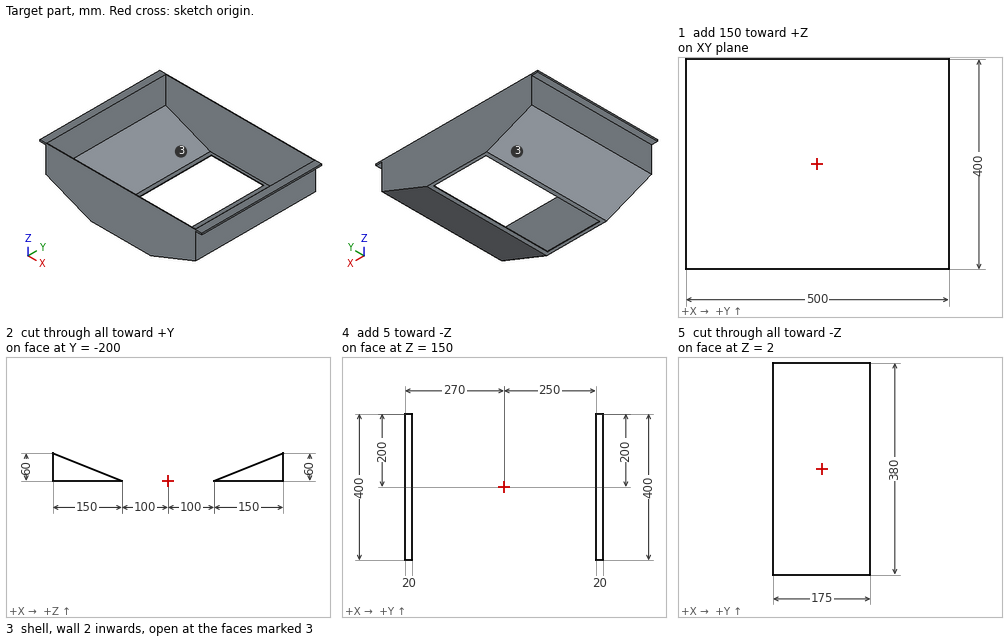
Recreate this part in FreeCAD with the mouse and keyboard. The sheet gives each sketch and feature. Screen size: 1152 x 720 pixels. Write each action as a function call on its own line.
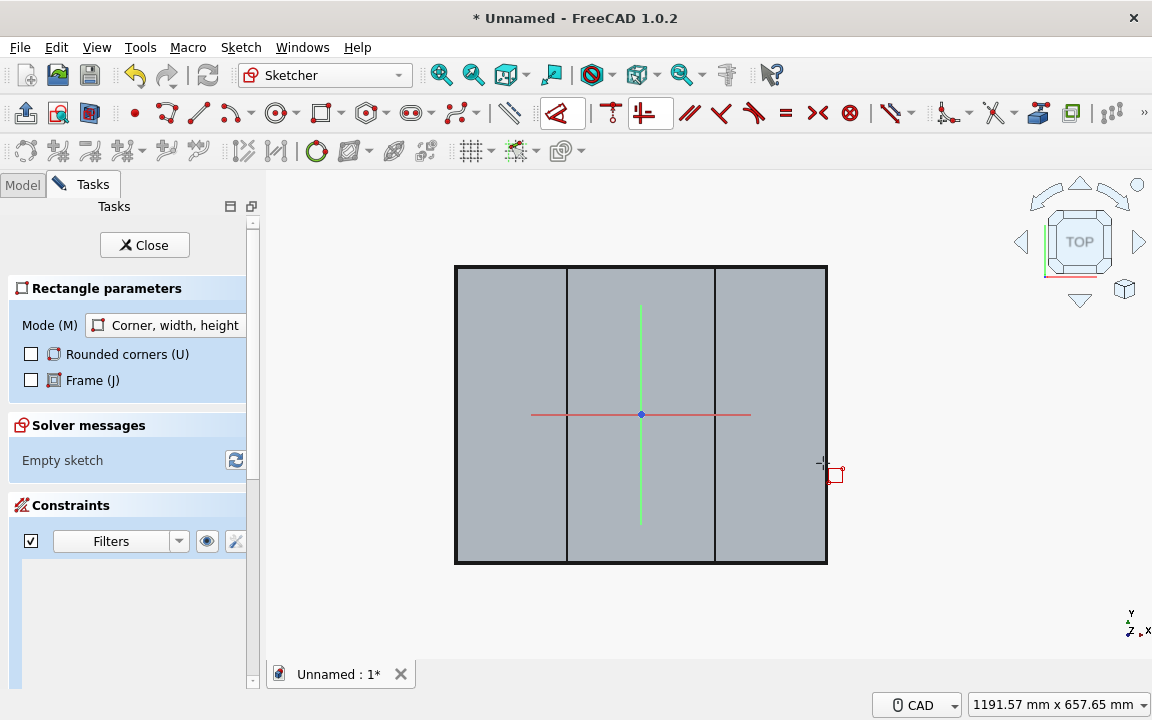
click(441, 266)
click(455, 564)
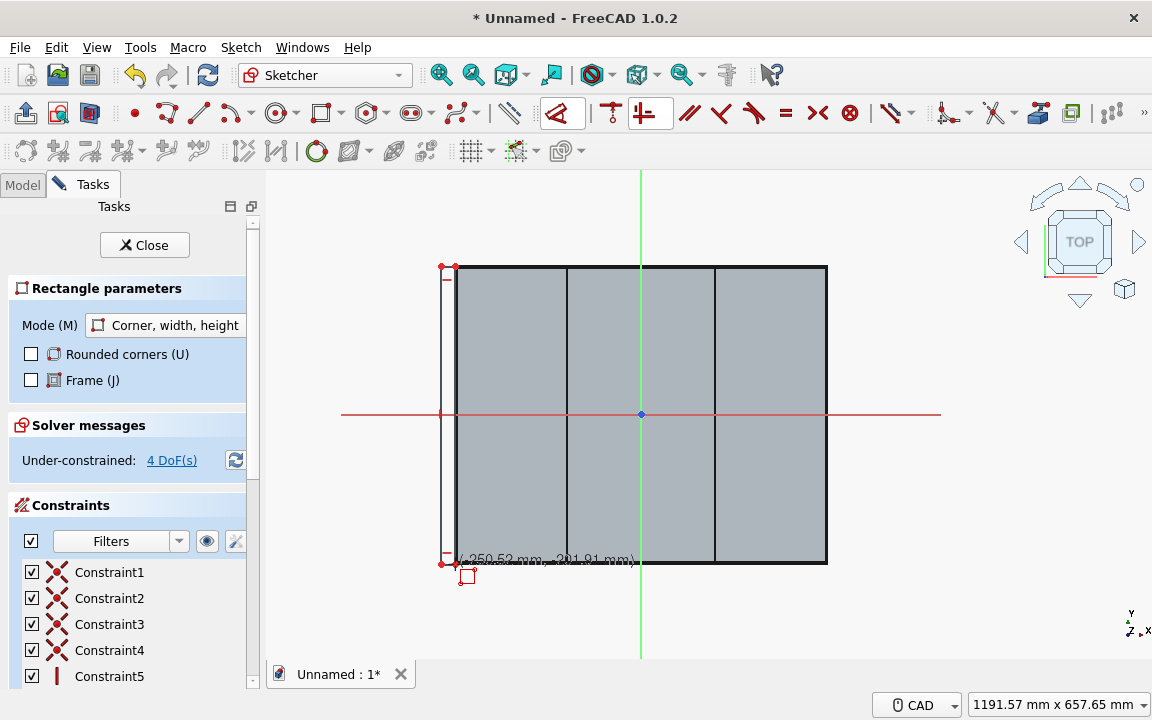
click(827, 266)
click(842, 564)
key(Escape)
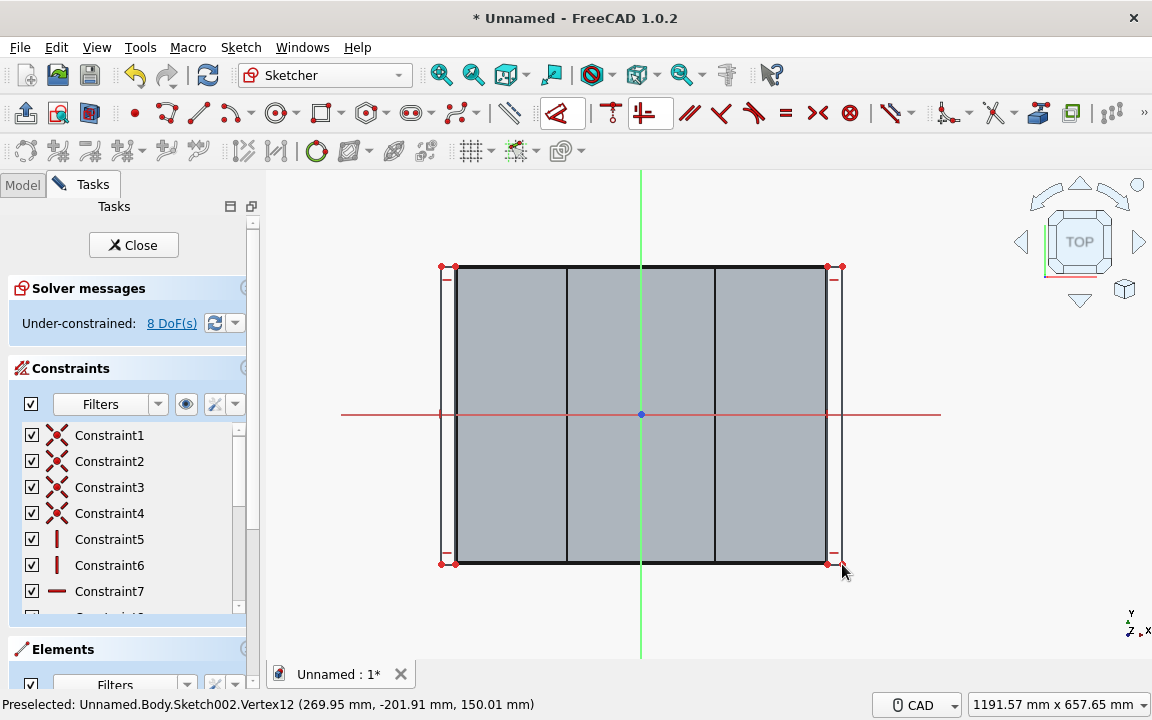
scroll(448, 565, up, 5)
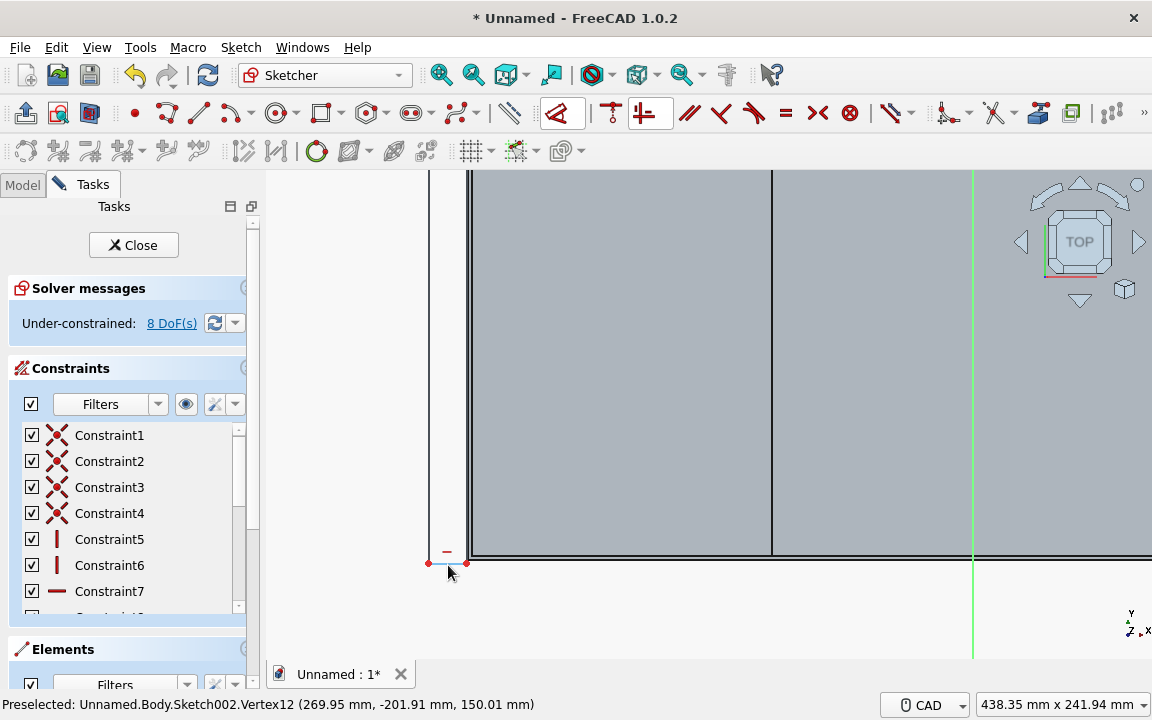
click(448, 564)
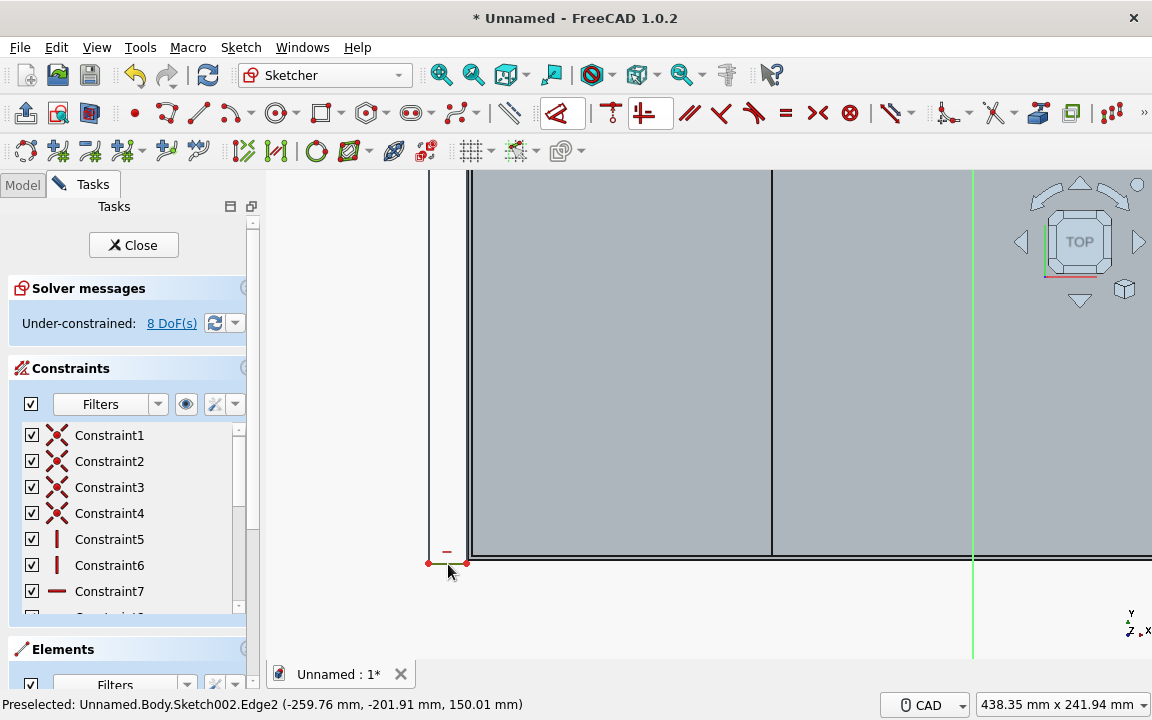
key(l)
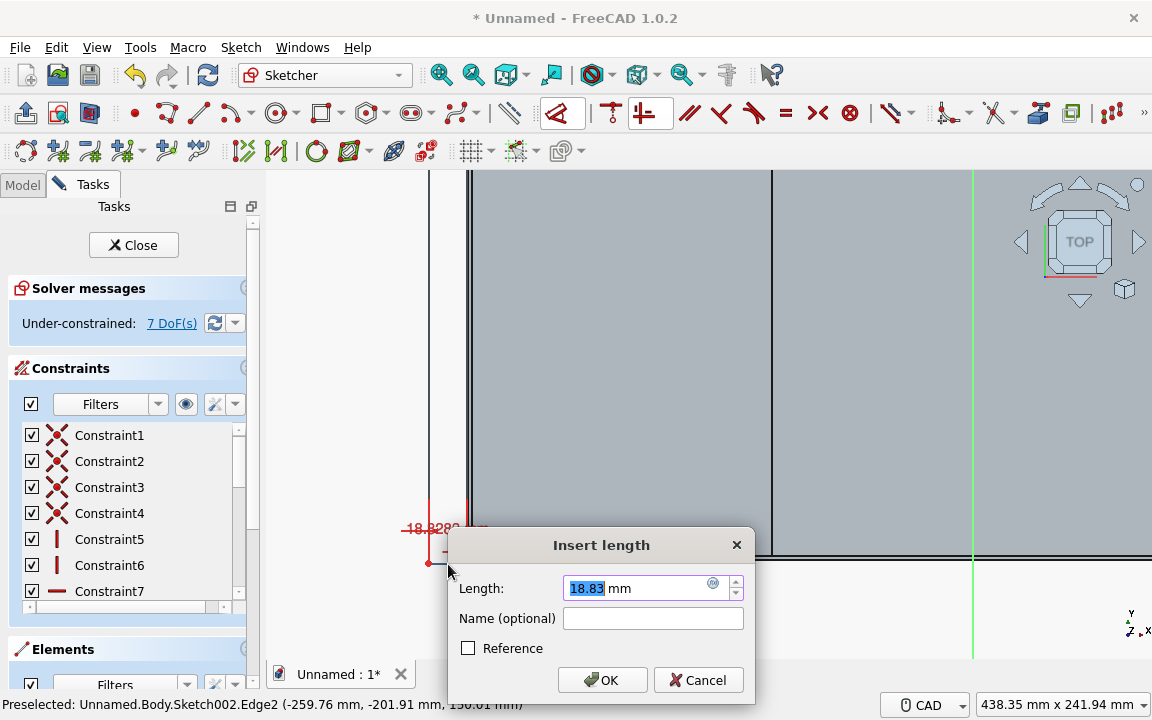
text(20)
key(Return)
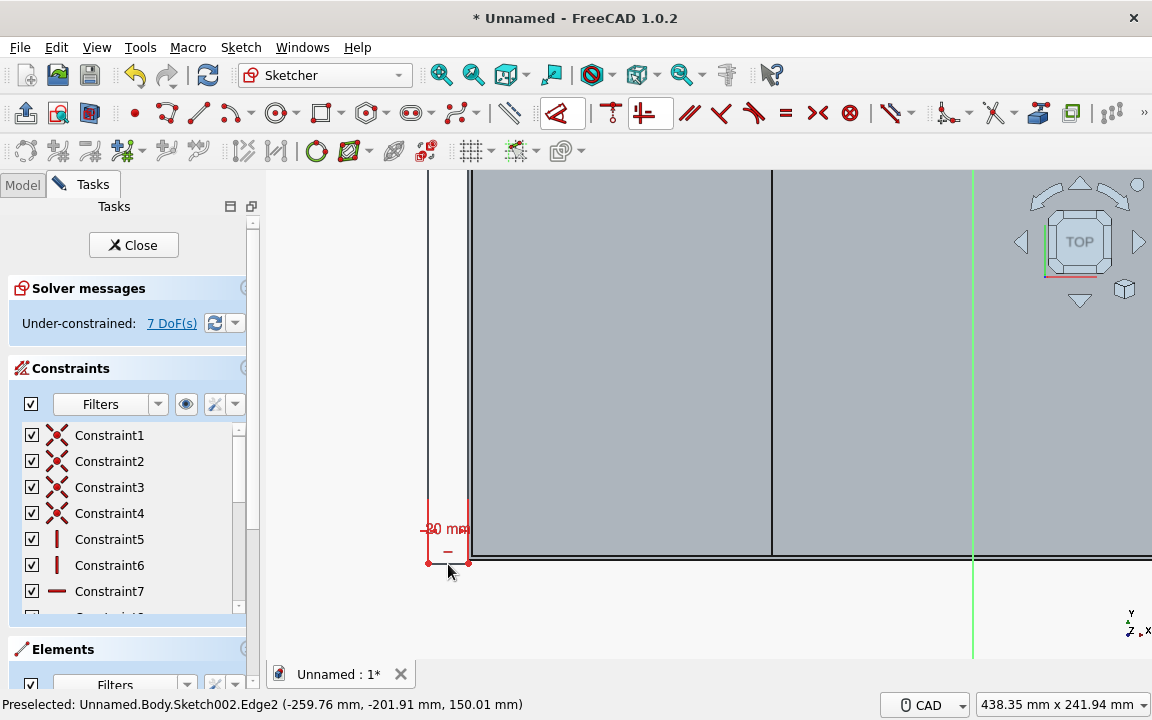
scroll(447, 565, down, 5)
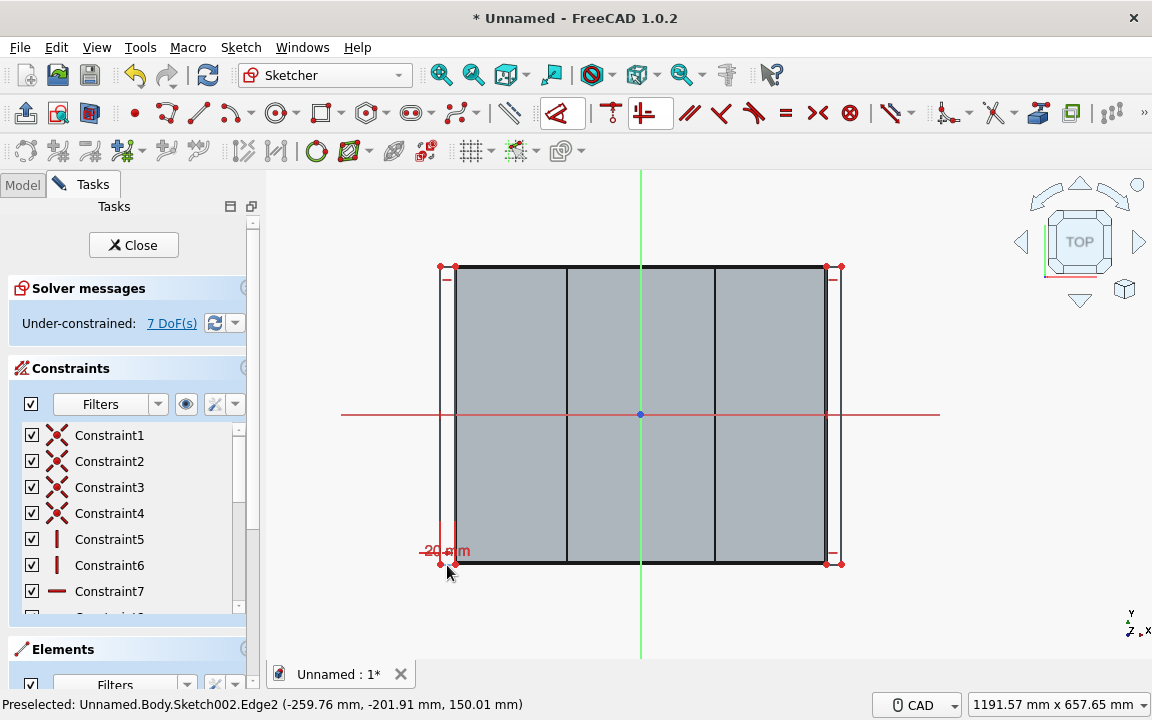
scroll(831, 565, up, 6)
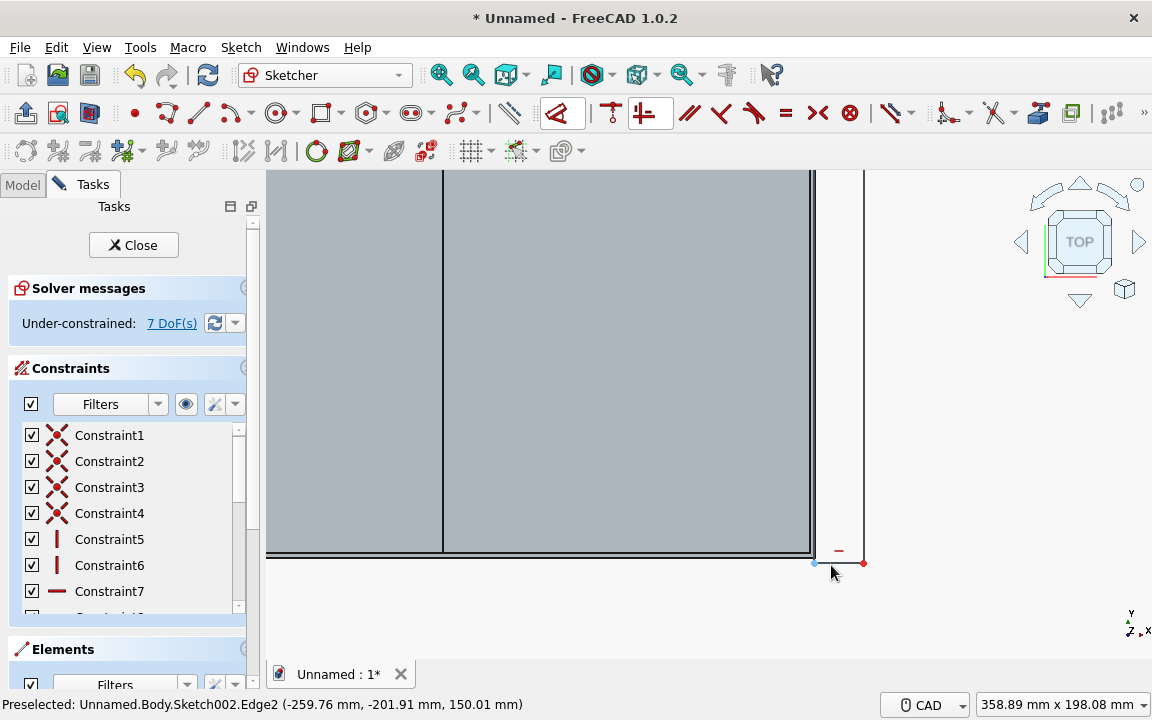
click(829, 563)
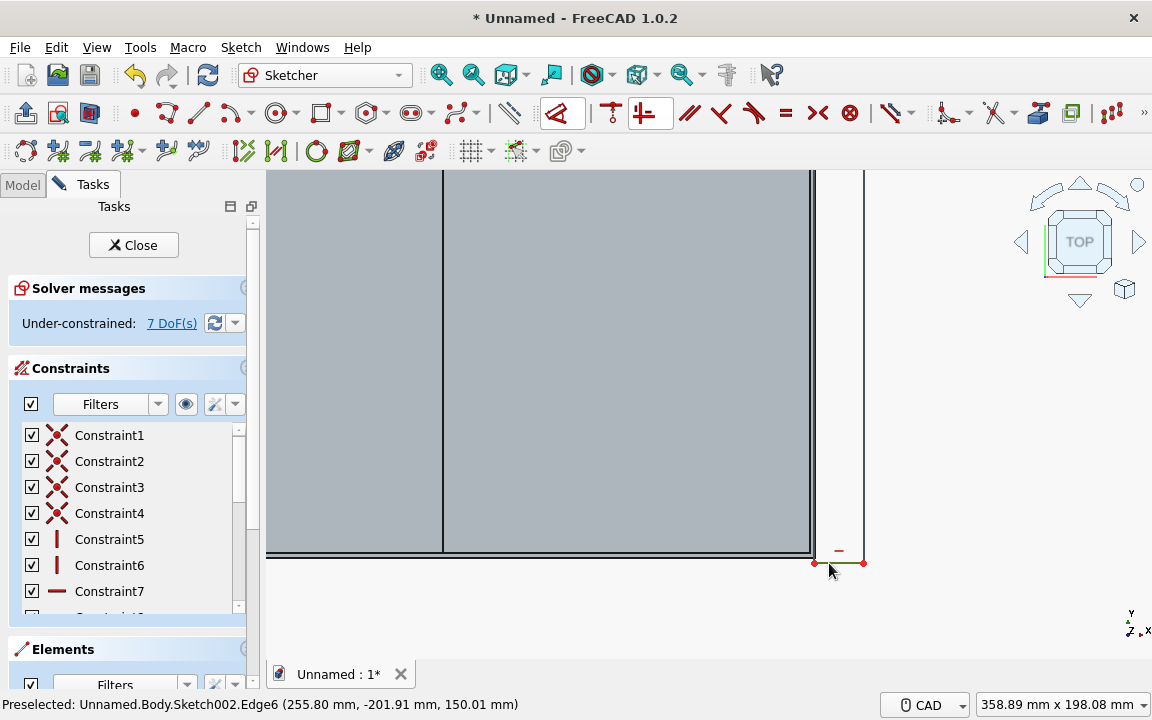
key(l)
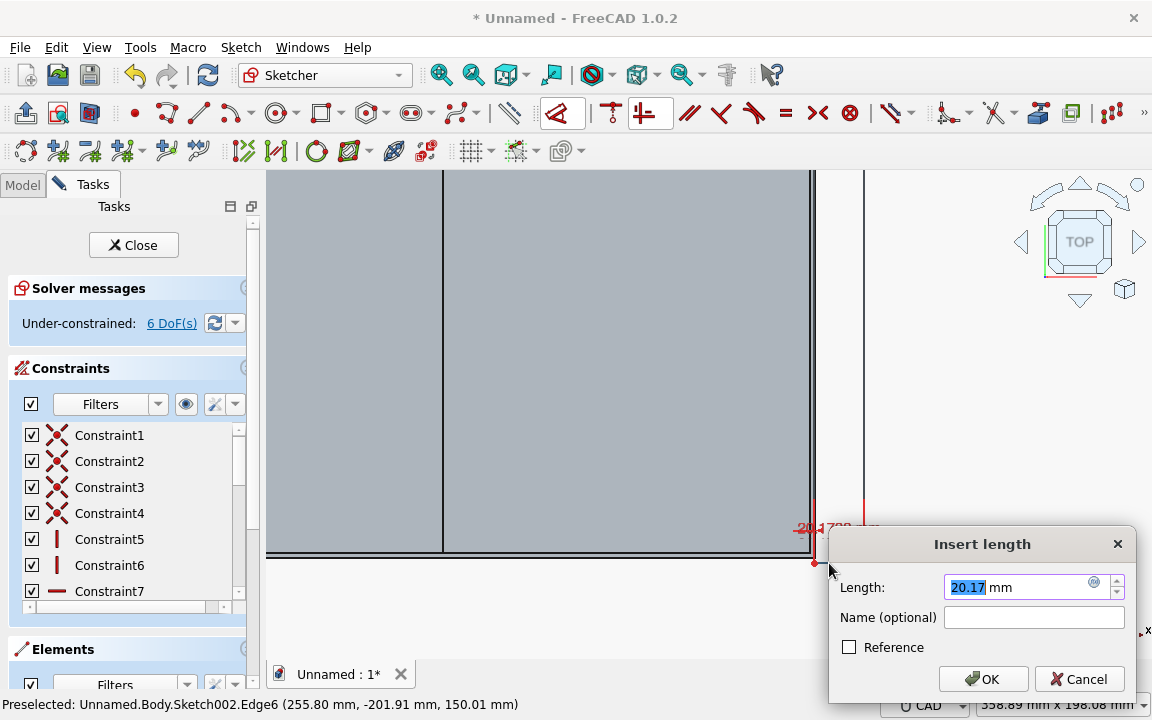
text(20)
key(Return)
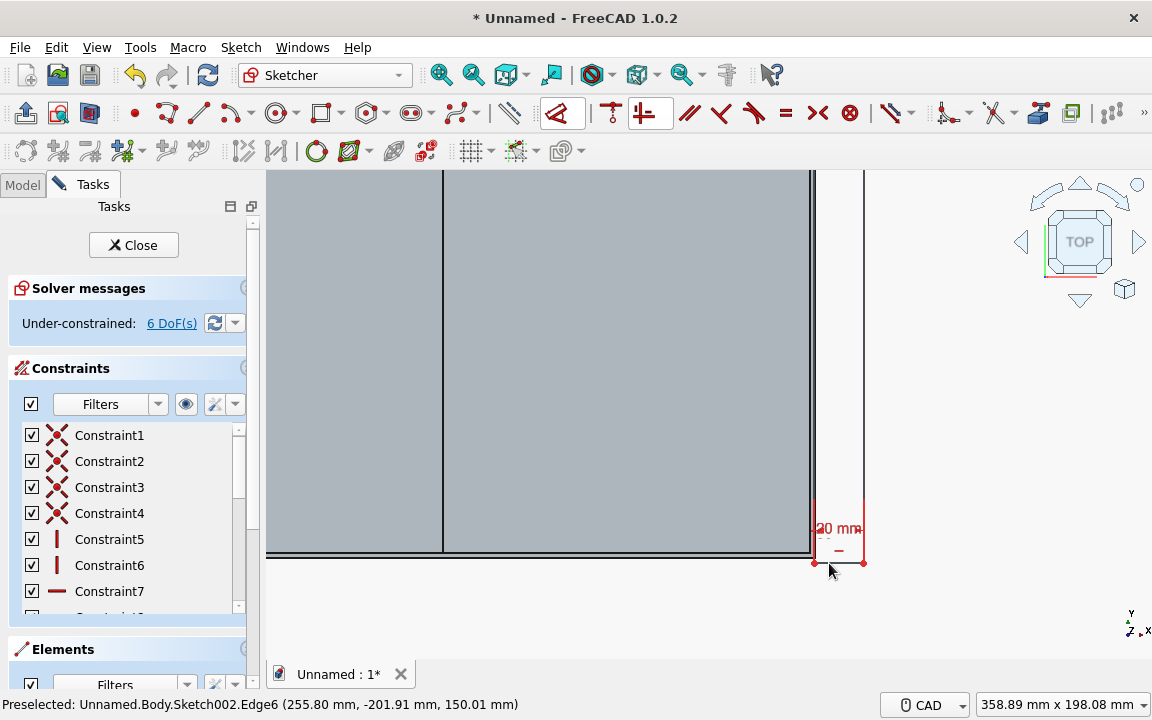
scroll(831, 565, down, 6)